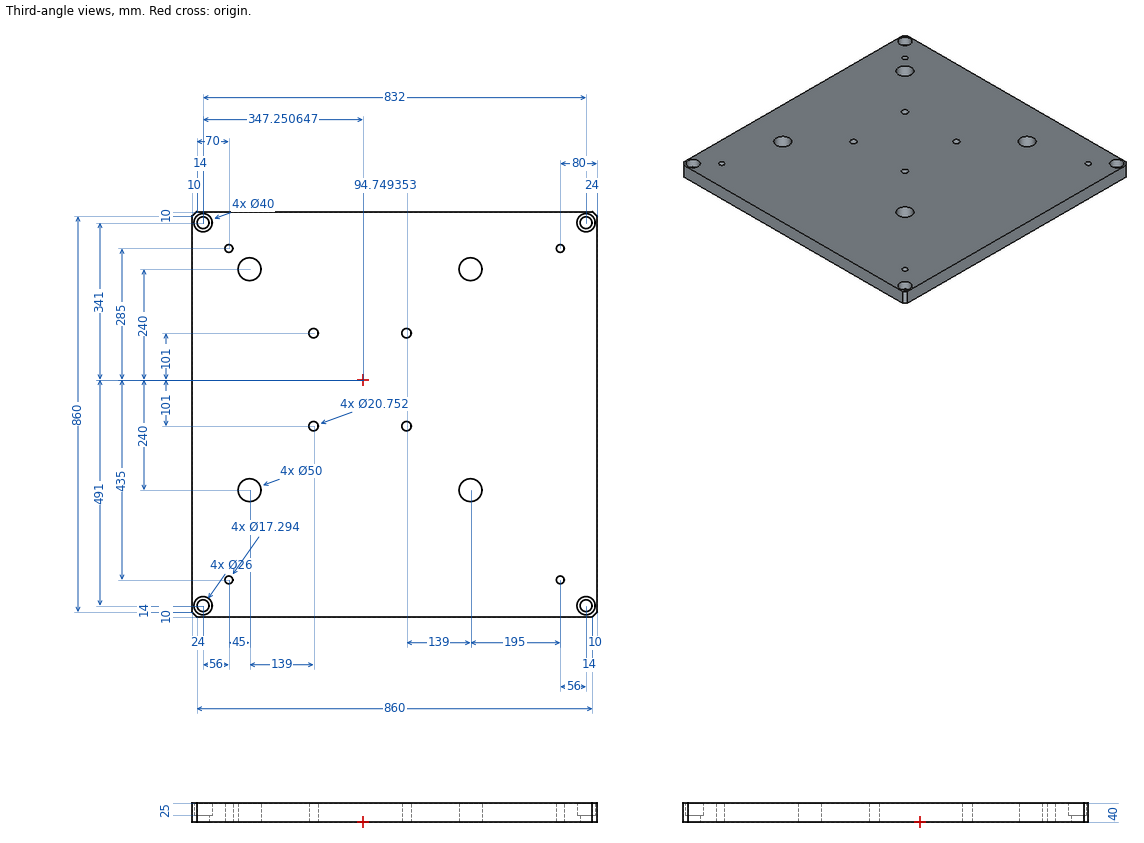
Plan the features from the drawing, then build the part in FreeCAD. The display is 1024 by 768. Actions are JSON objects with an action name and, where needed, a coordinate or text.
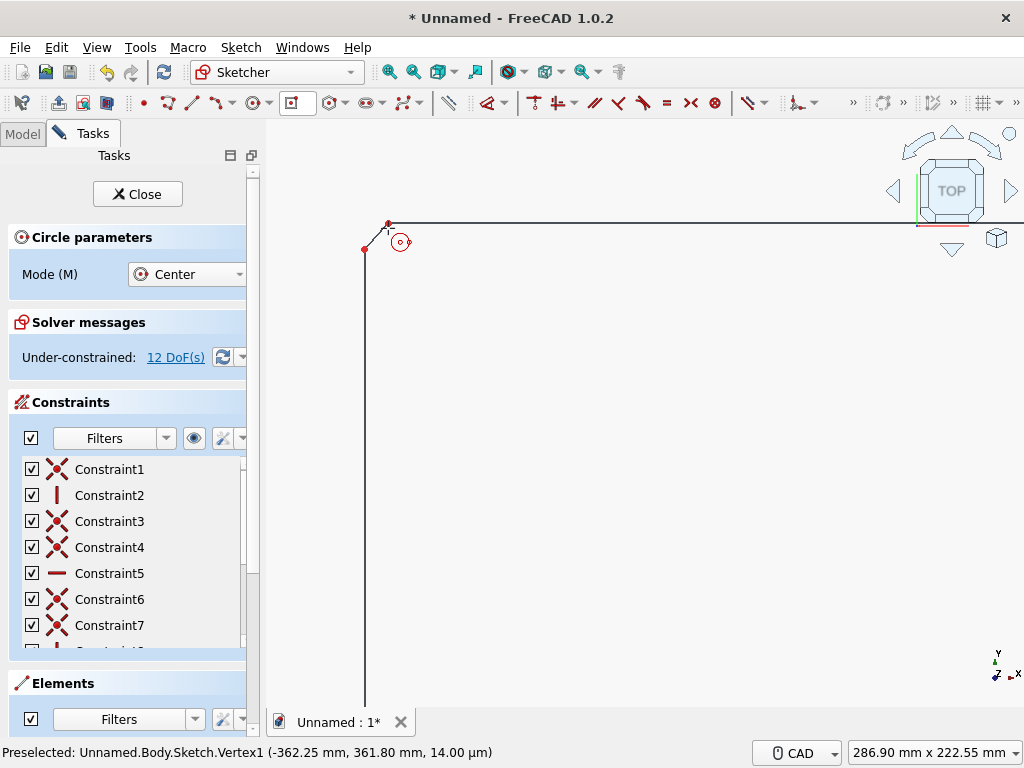
{"action": "scroll", "coordinate": [388, 221], "scroll_direction": "down", "scroll_amount": 9}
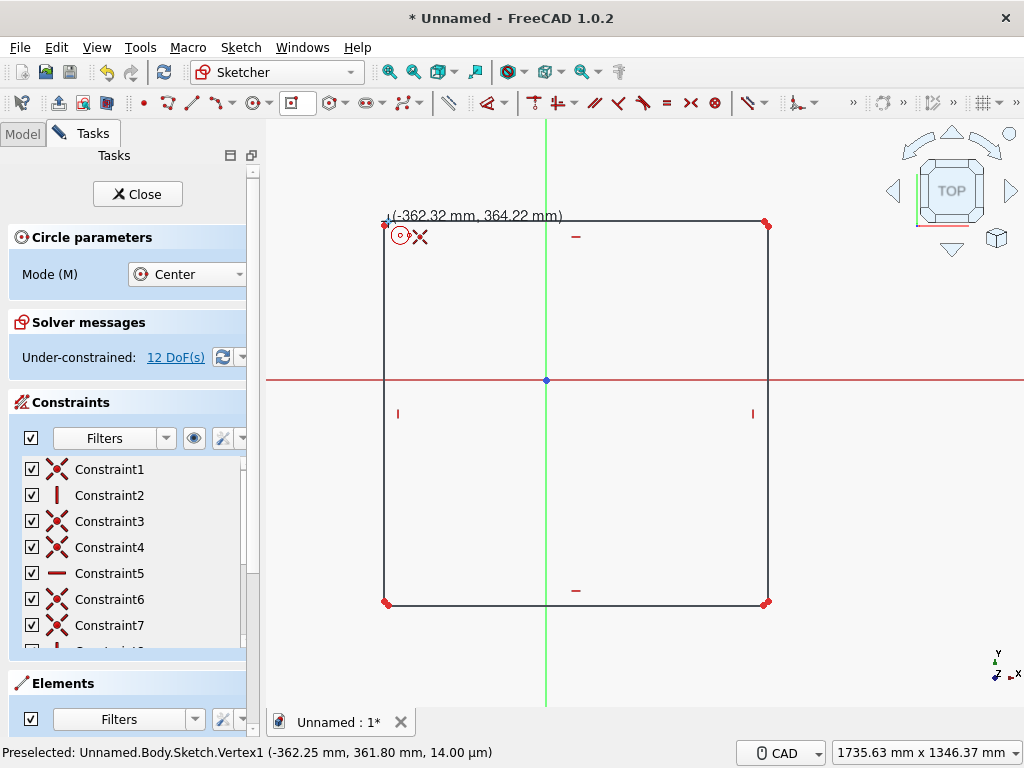
{"action": "scroll", "coordinate": [395, 595], "scroll_direction": "up", "scroll_amount": 7}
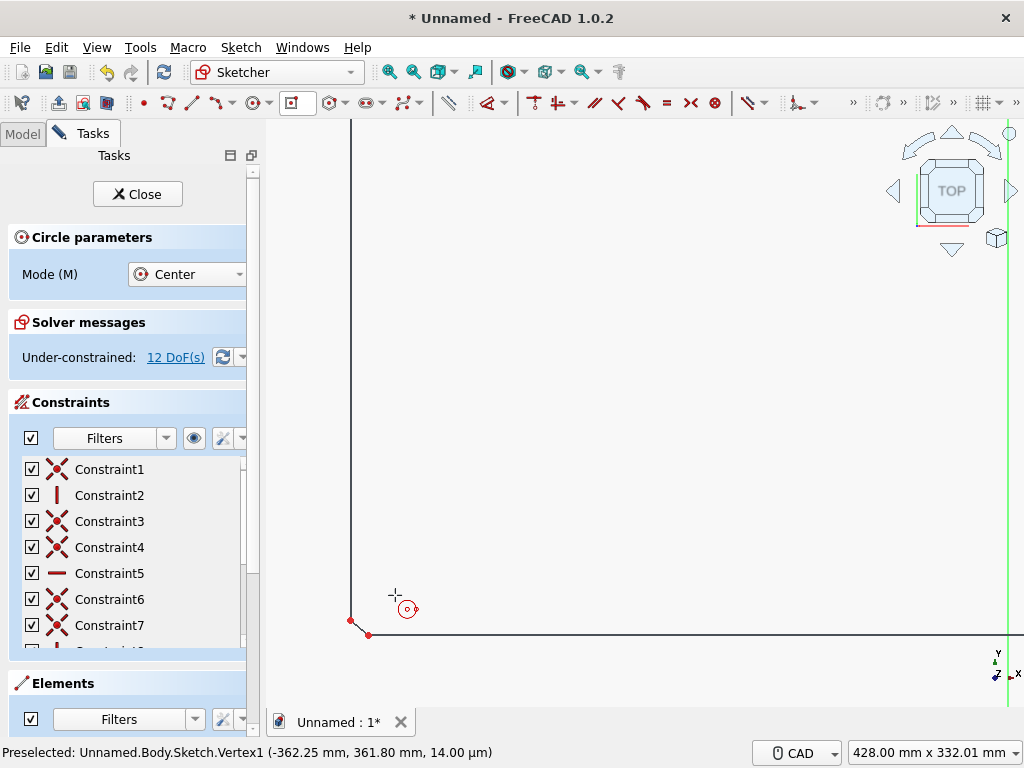
{"action": "left_click", "coordinate": [393, 592]}
{"action": "left_click", "coordinate": [410, 575]}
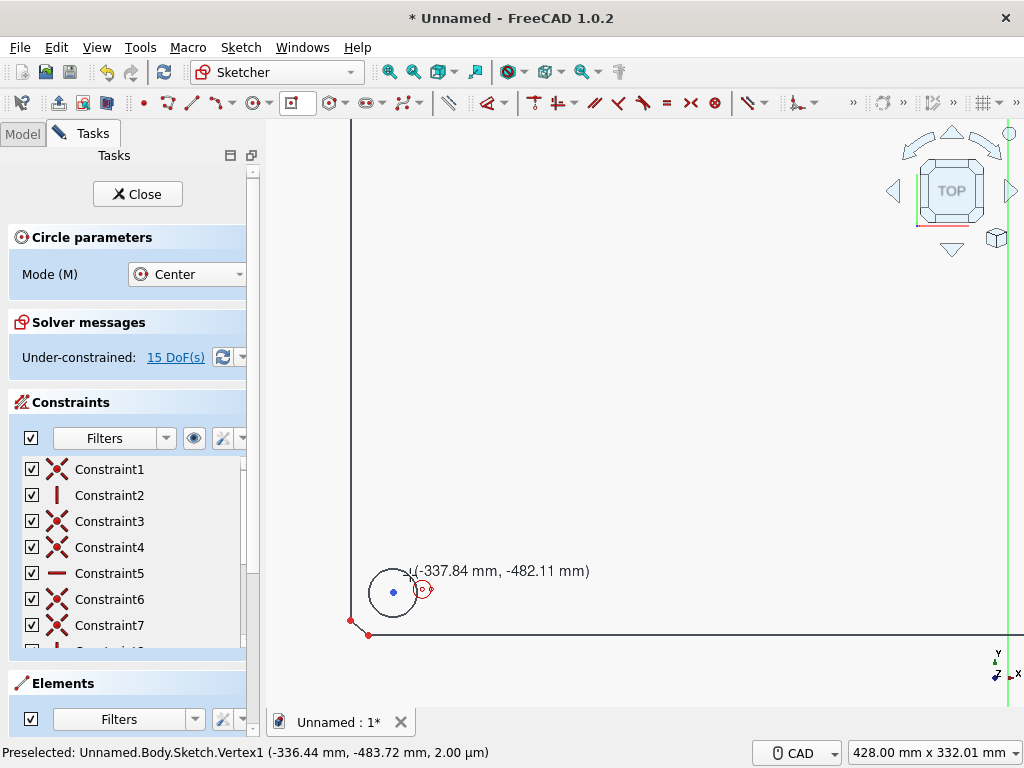
{"action": "scroll", "coordinate": [493, 493], "scroll_direction": "up", "scroll_amount": 2}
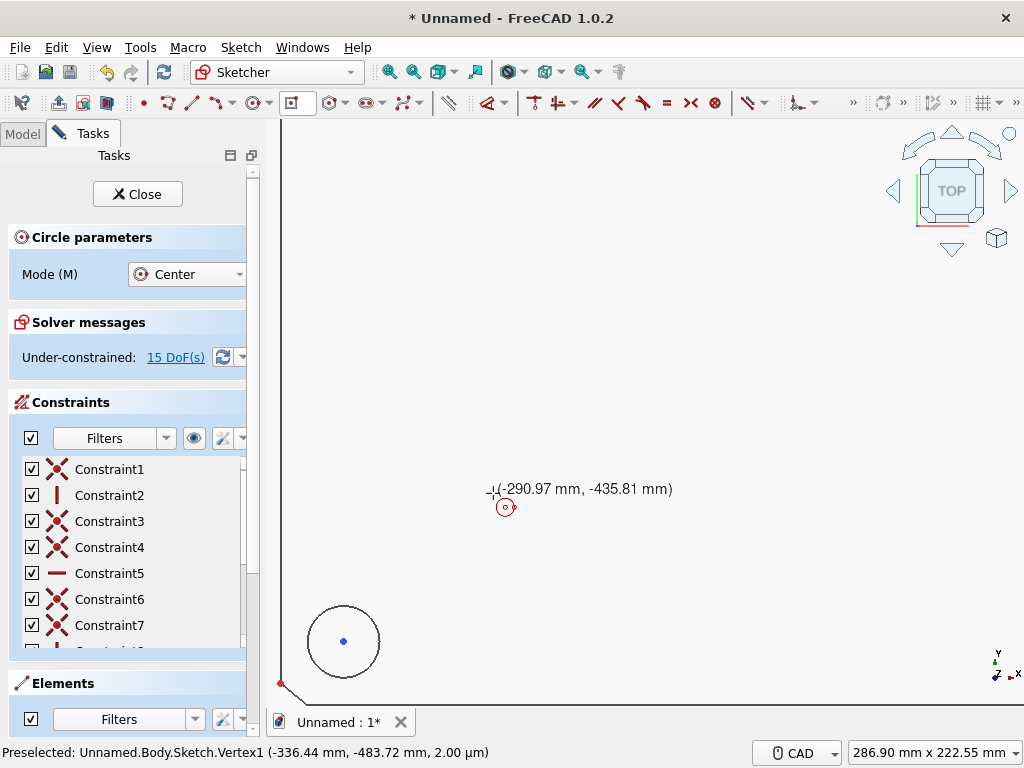
{"action": "scroll", "coordinate": [405, 586], "scroll_direction": "down", "scroll_amount": 9}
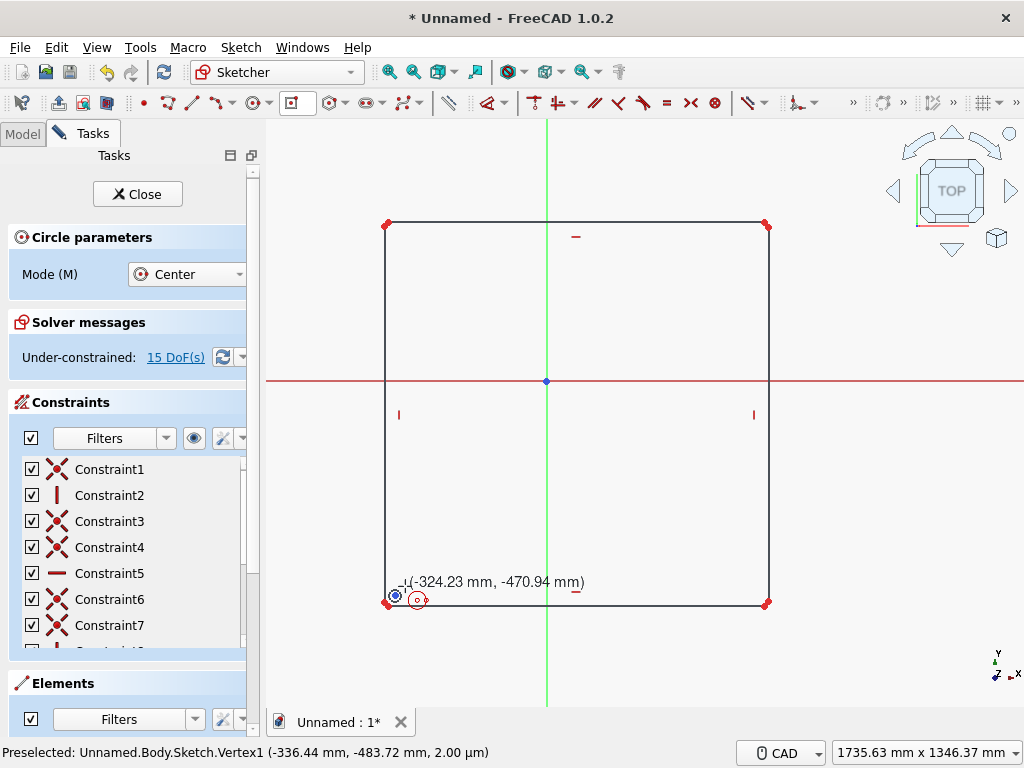
{"action": "left_click", "coordinate": [420, 571]}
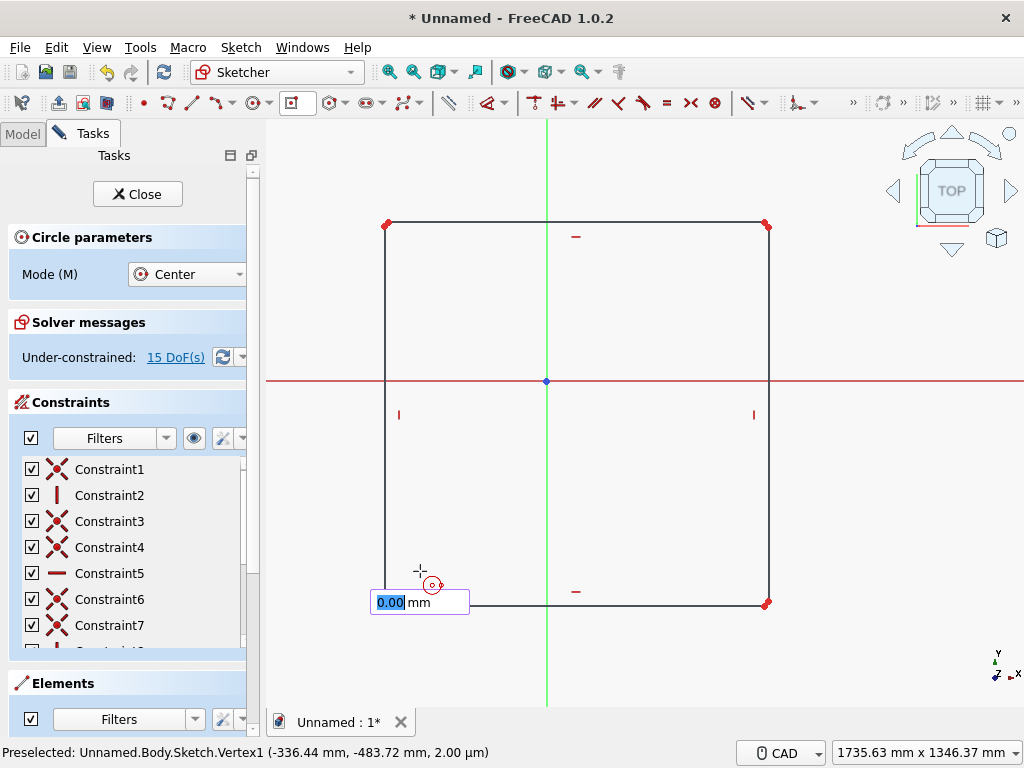
{"action": "scroll", "coordinate": [422, 568], "scroll_direction": "up", "scroll_amount": 8}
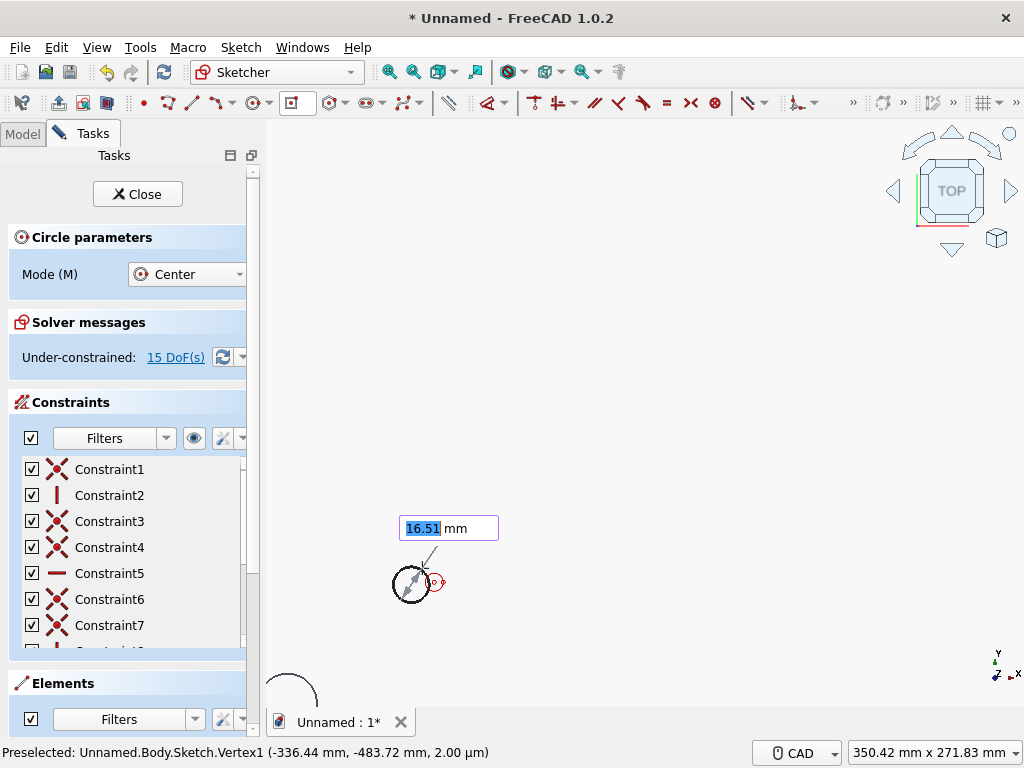
{"action": "left_click", "coordinate": [422, 567]}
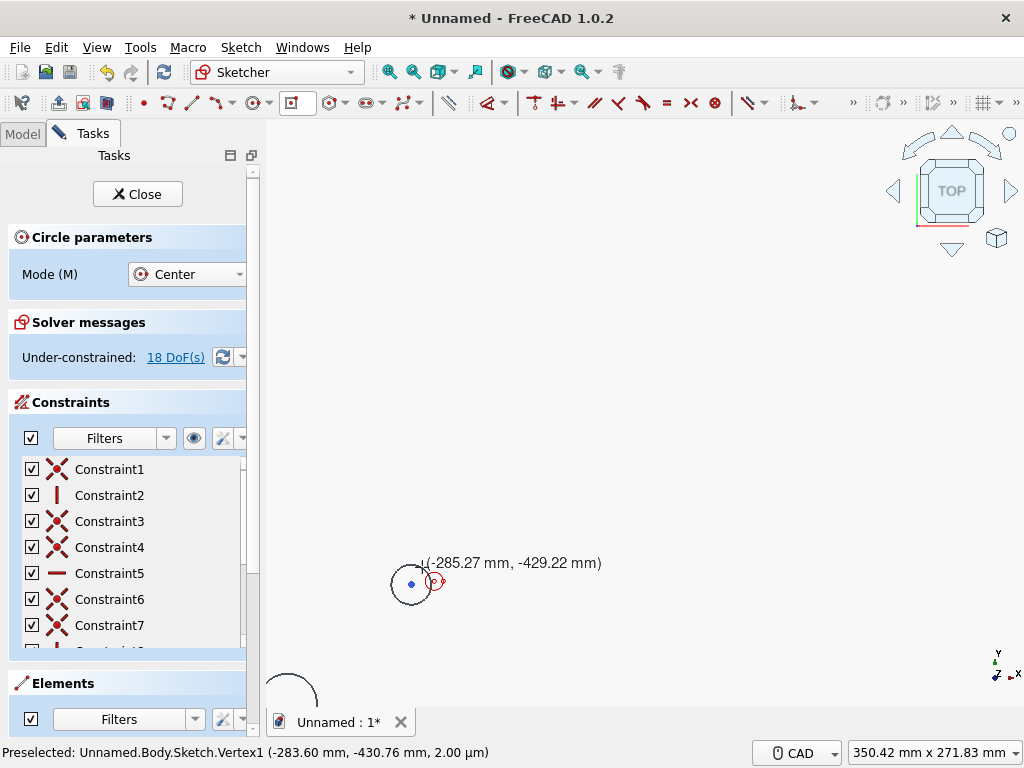
{"action": "scroll", "coordinate": [422, 568], "scroll_direction": "down", "scroll_amount": 8}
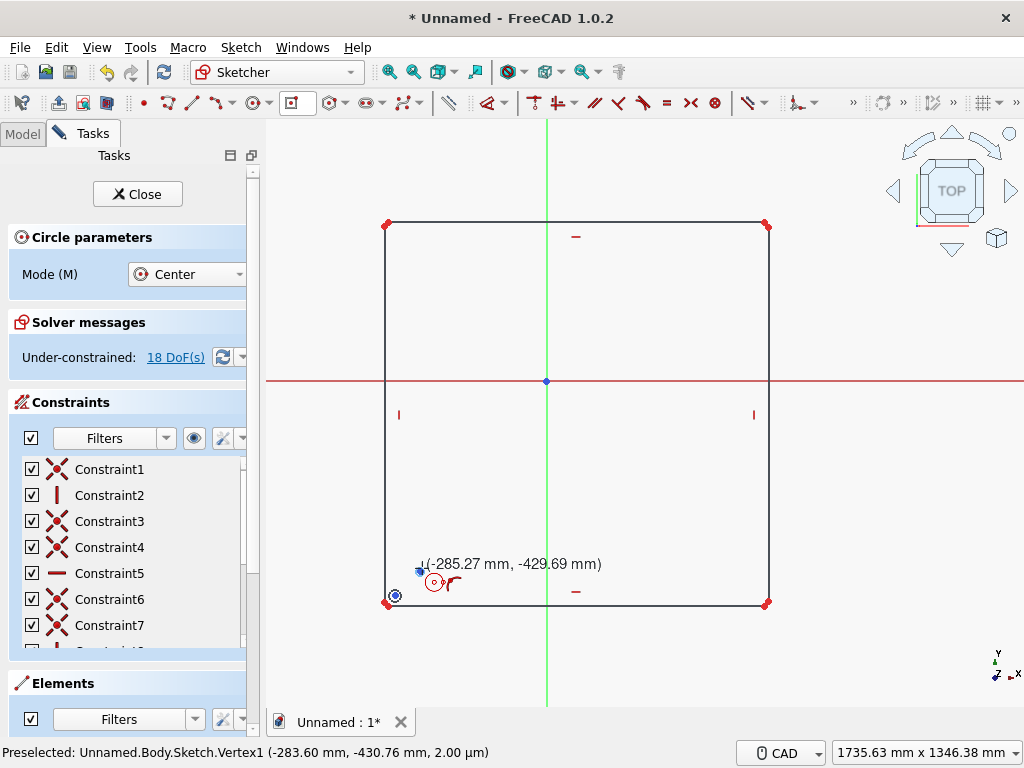
{"action": "left_click", "coordinate": [439, 486]}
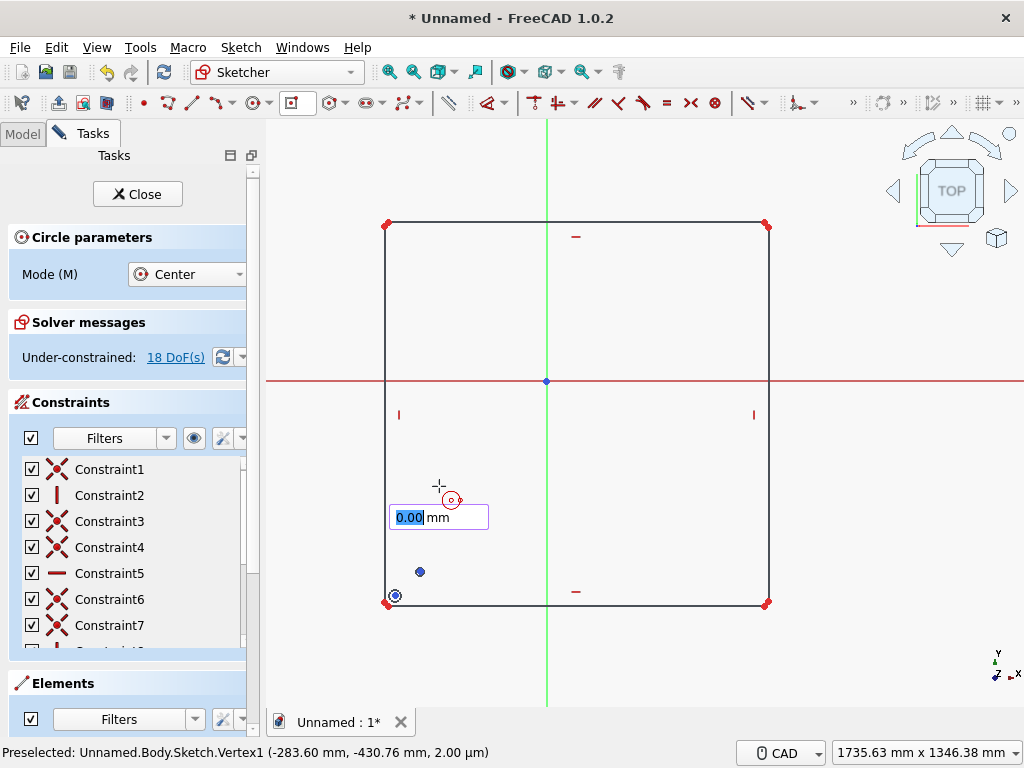
{"action": "scroll", "coordinate": [447, 478], "scroll_direction": "up", "scroll_amount": 2}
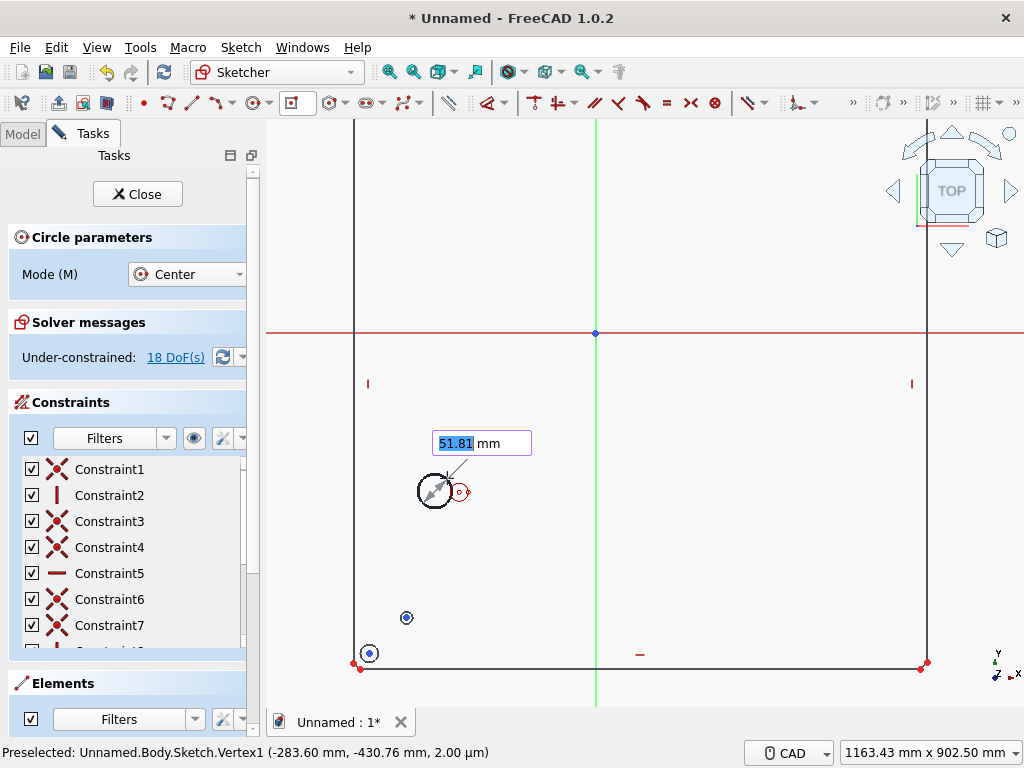
{"action": "left_click", "coordinate": [447, 478]}